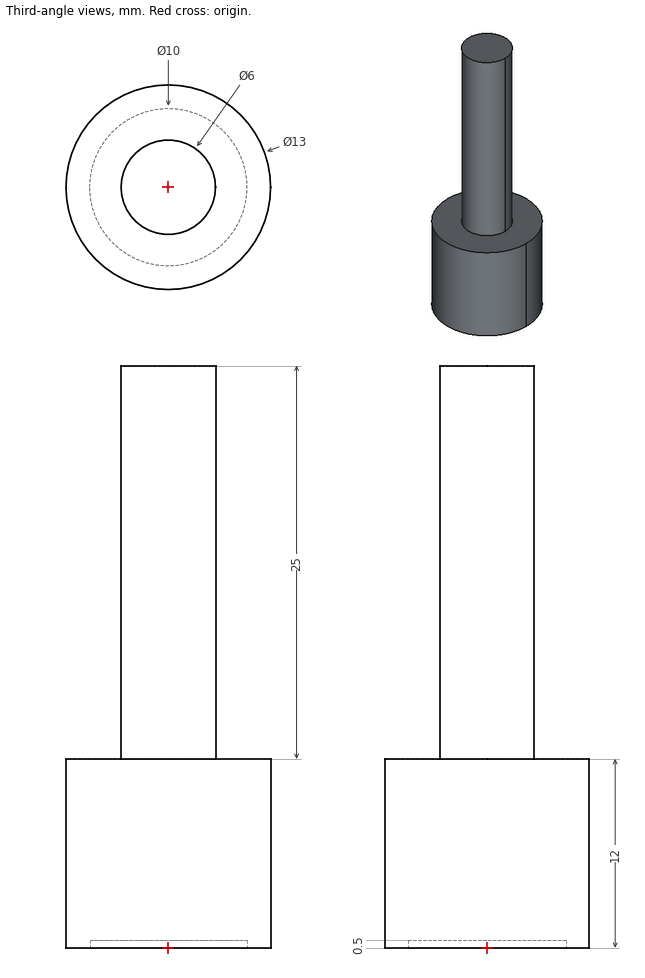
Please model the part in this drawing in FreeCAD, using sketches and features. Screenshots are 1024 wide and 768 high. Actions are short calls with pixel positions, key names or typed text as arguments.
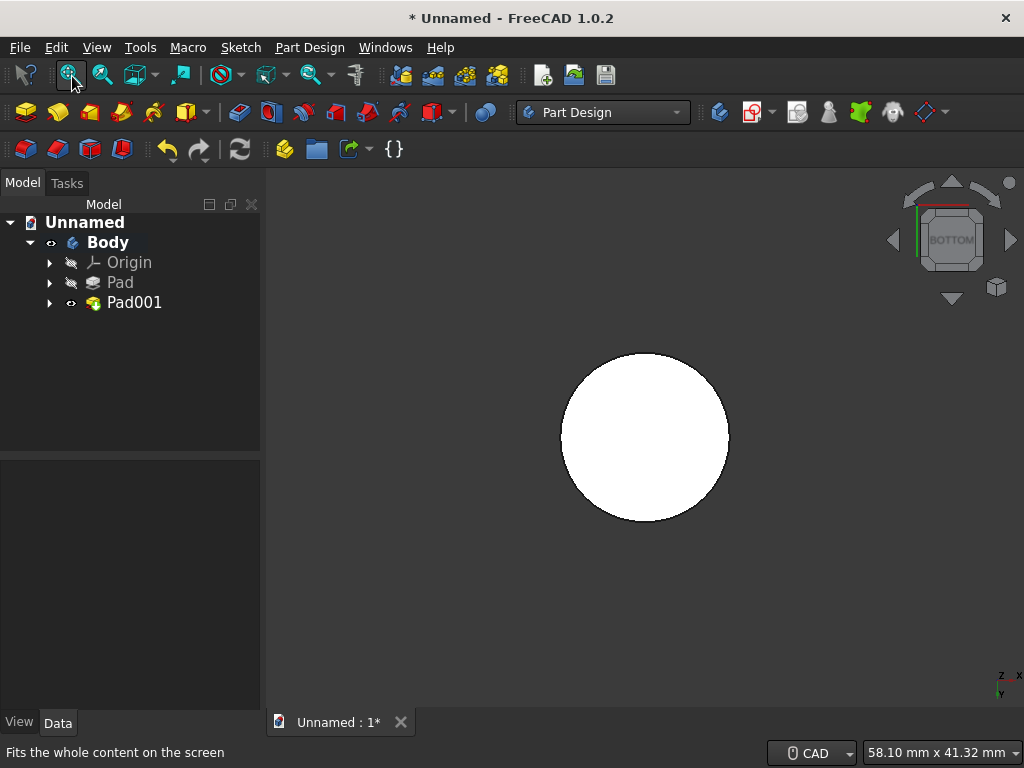
click(645, 436)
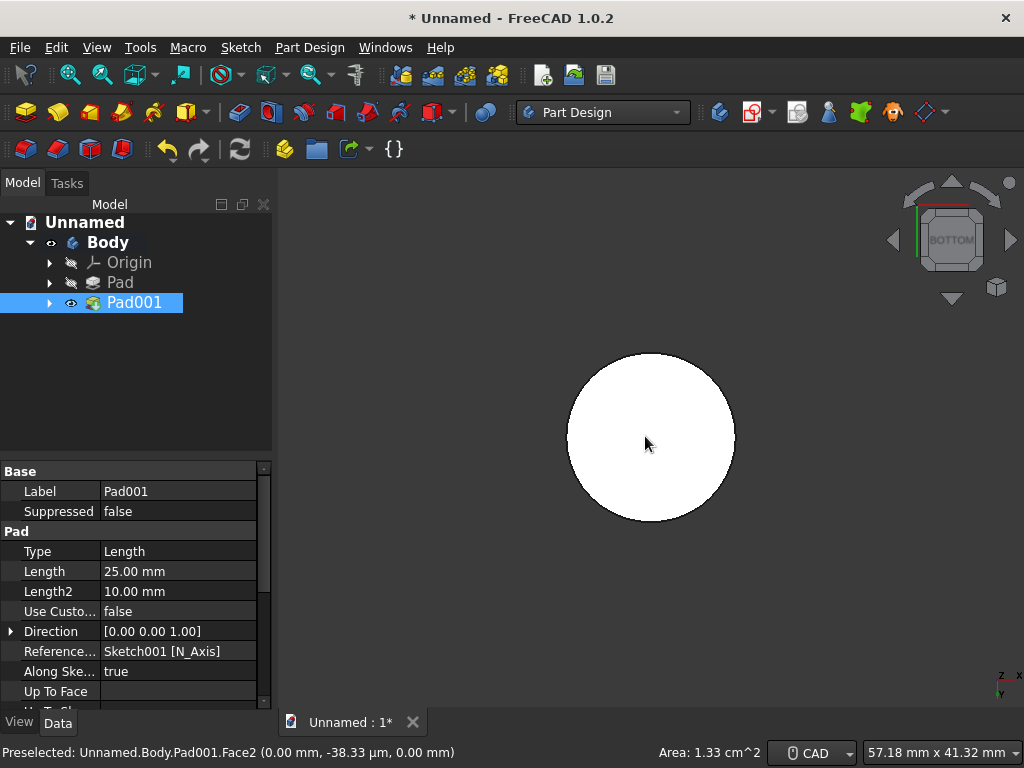
click(752, 112)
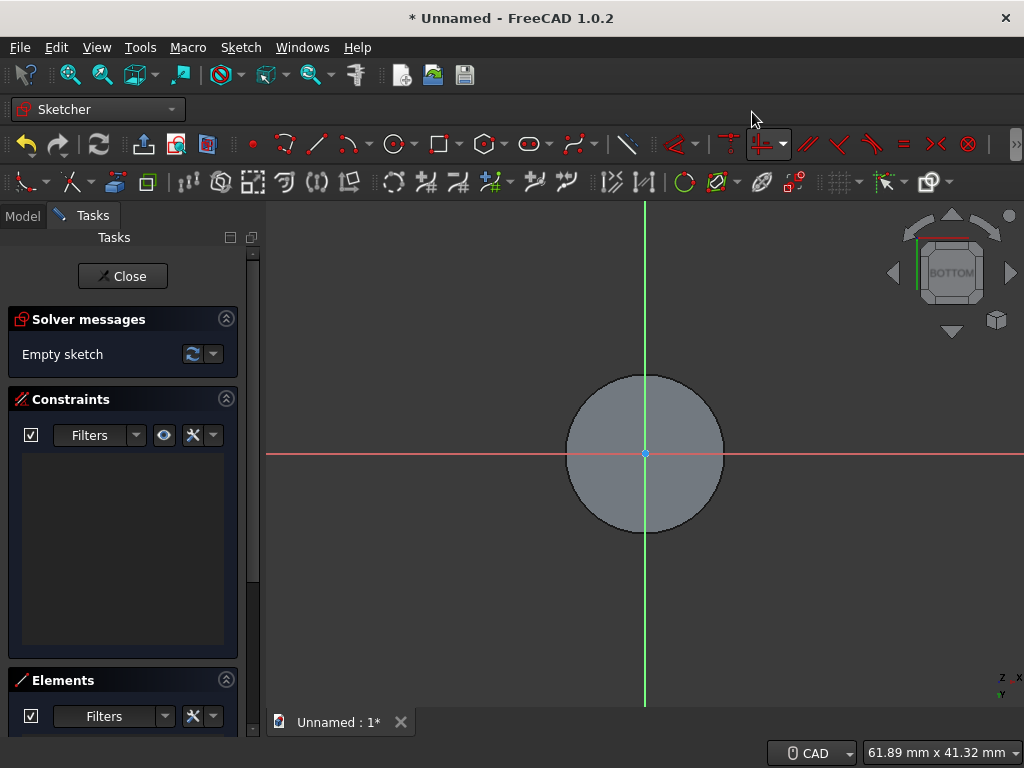
scroll(685, 454, up, 5)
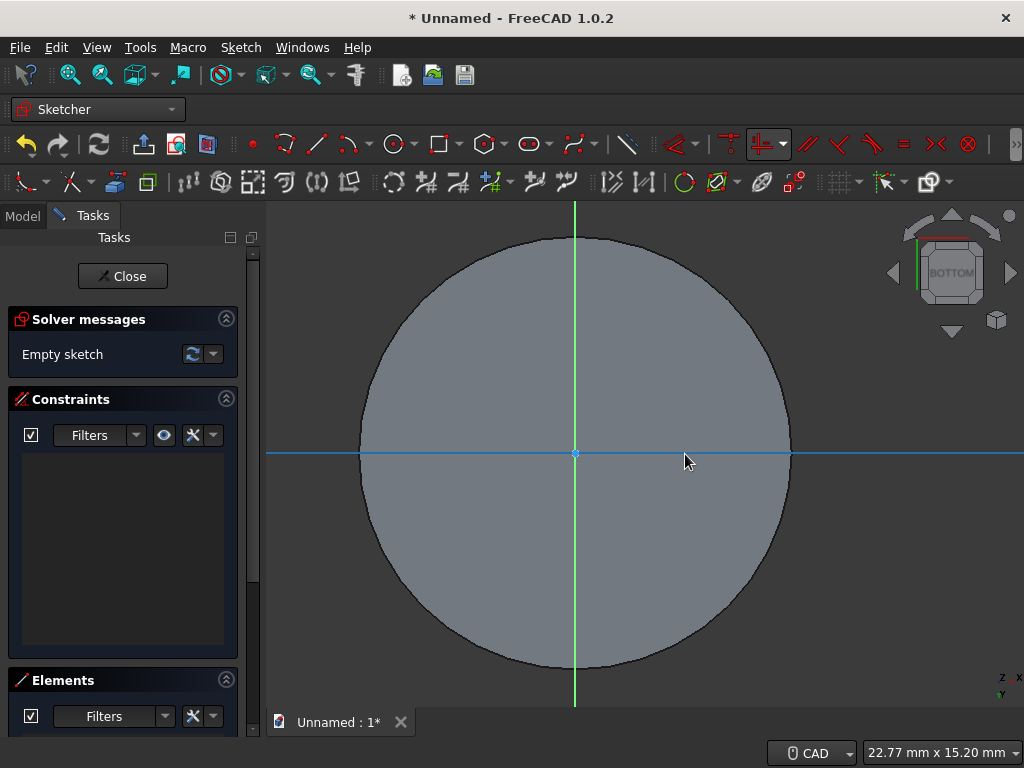
click(394, 144)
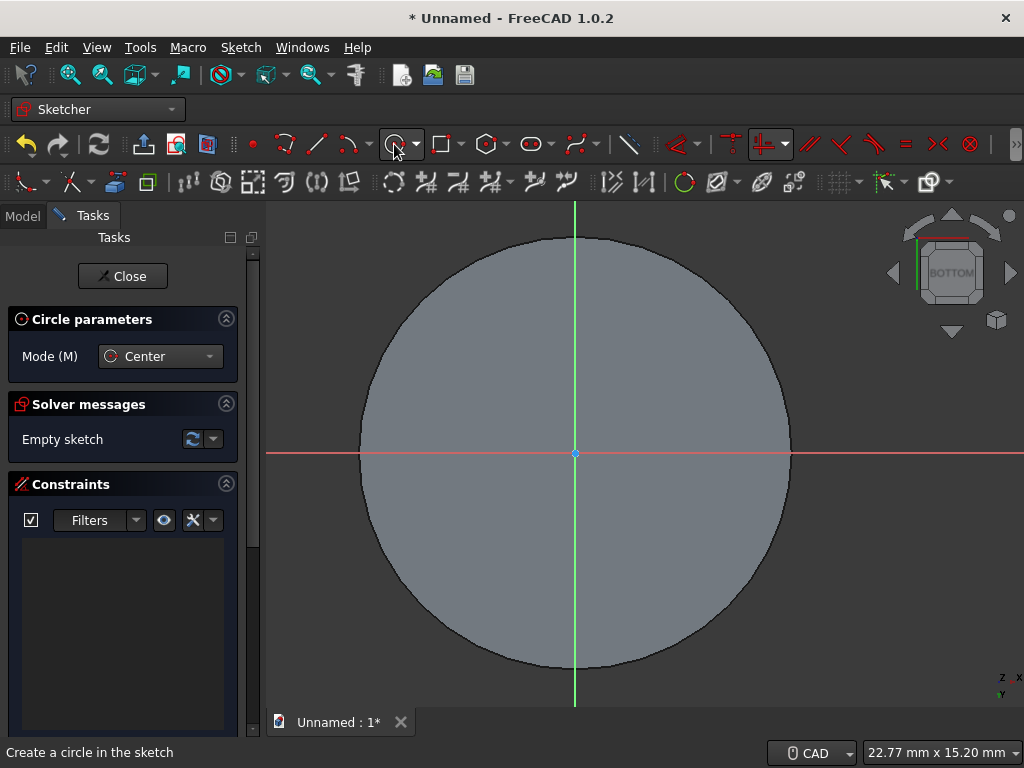
click(575, 453)
move(693, 335)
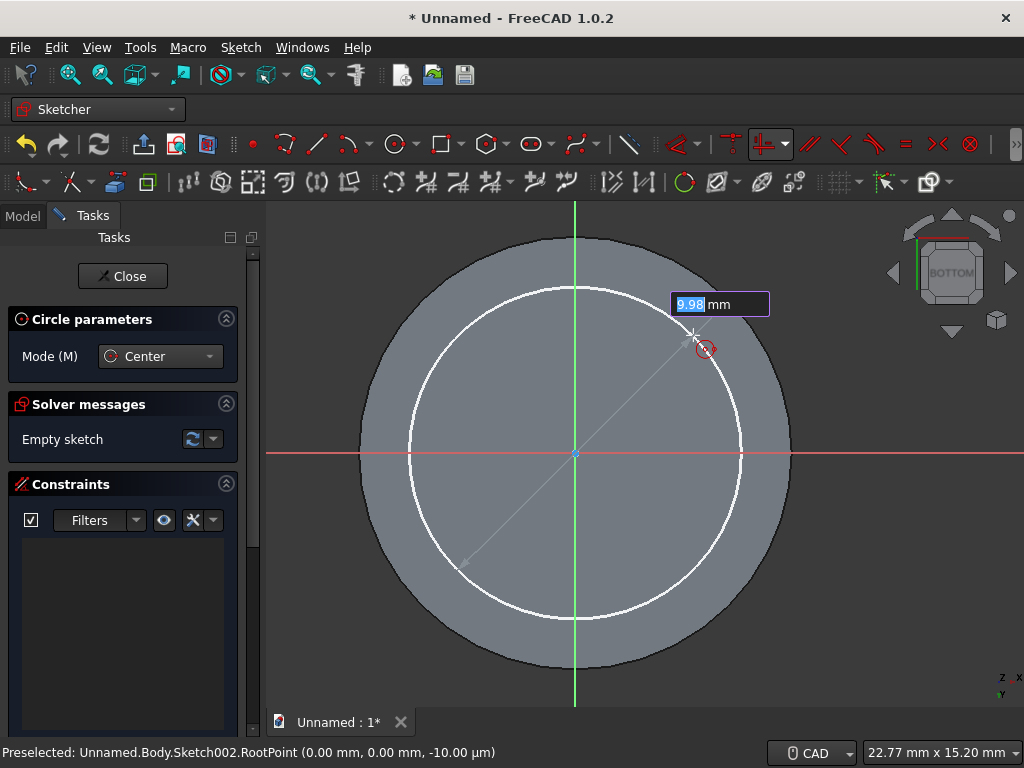
text(10)
key(Return)
key(Escape)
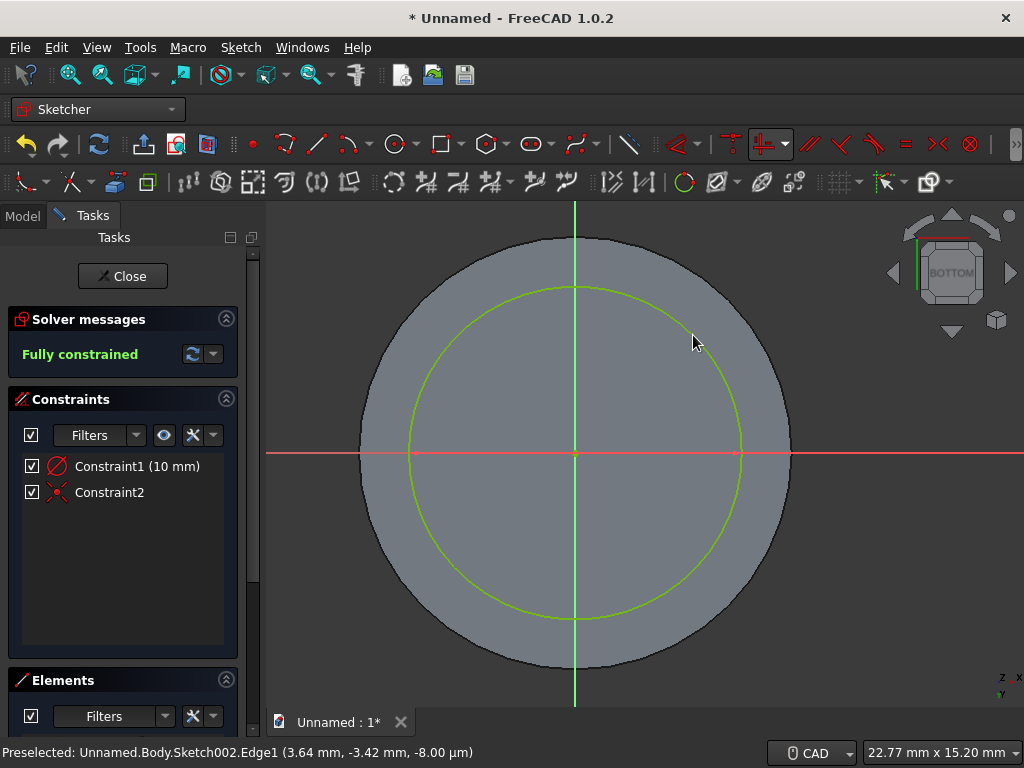
click(123, 276)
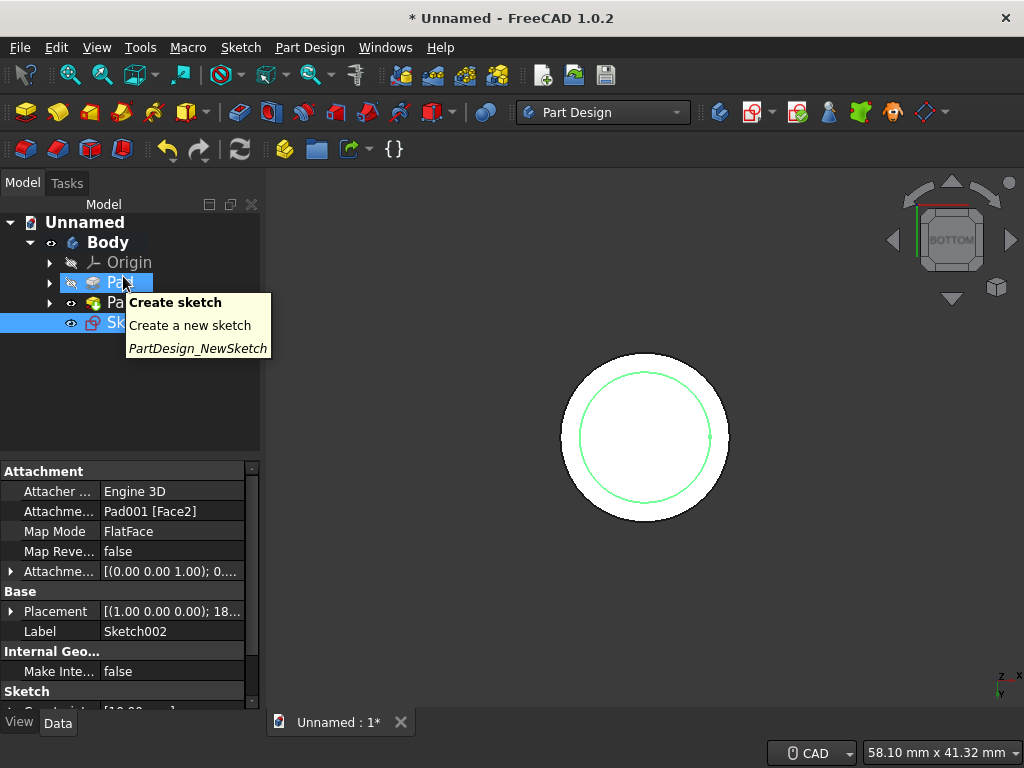
click(240, 112)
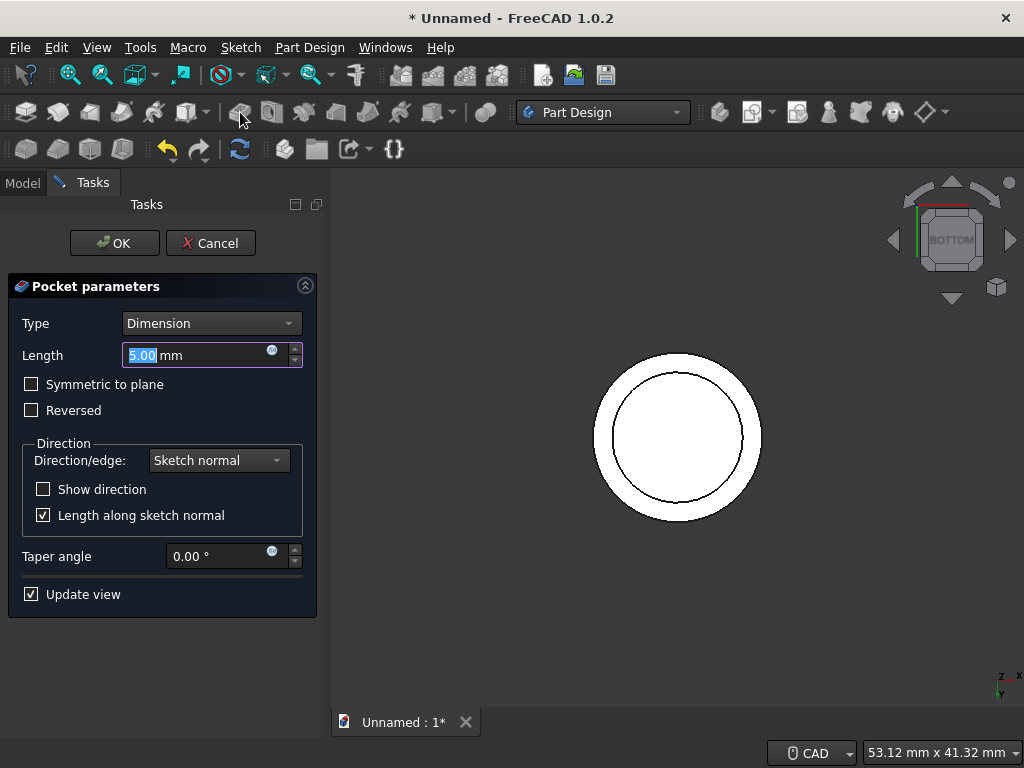
text(0.5)
key(Tab)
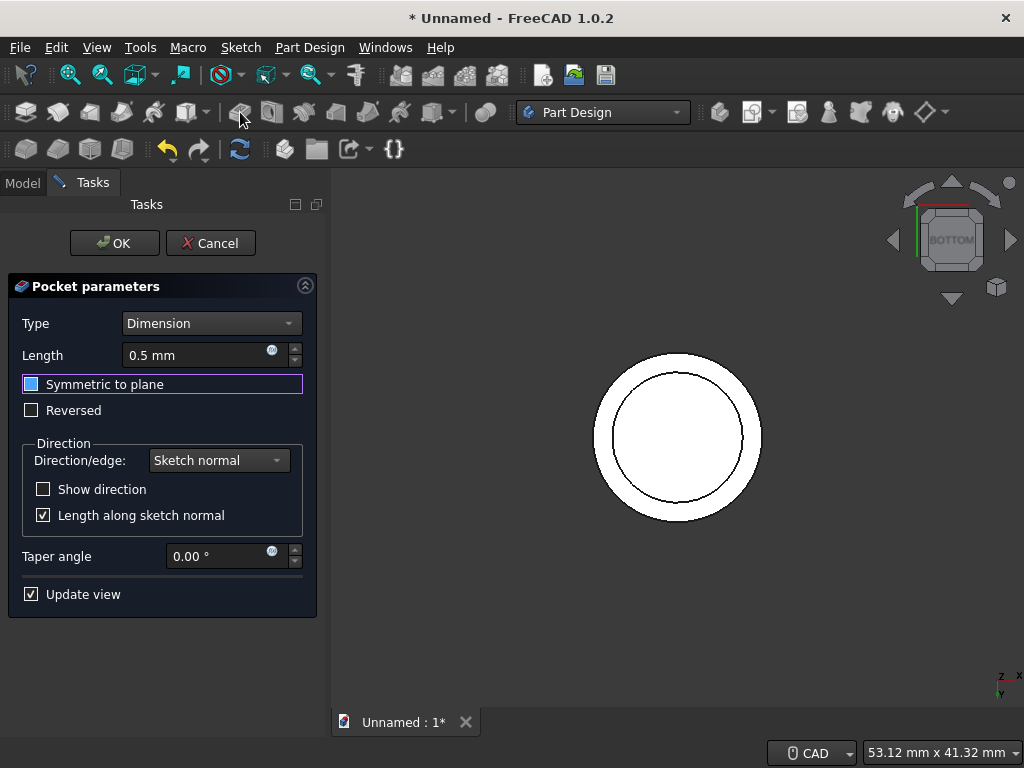
click(115, 243)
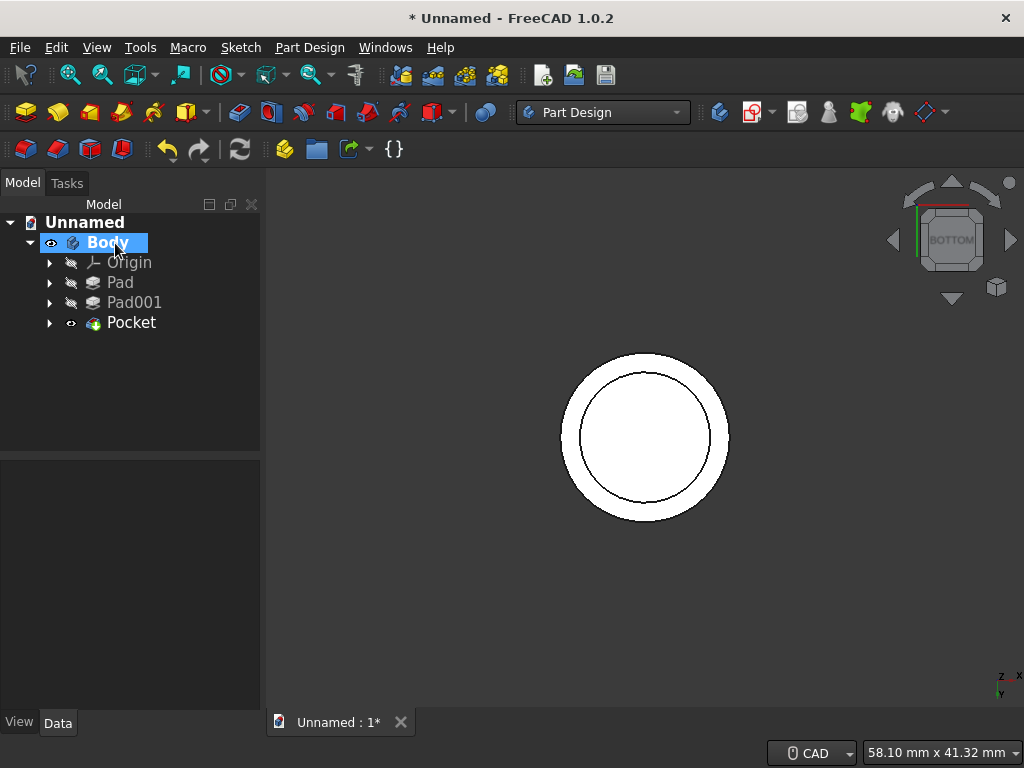
key(0)